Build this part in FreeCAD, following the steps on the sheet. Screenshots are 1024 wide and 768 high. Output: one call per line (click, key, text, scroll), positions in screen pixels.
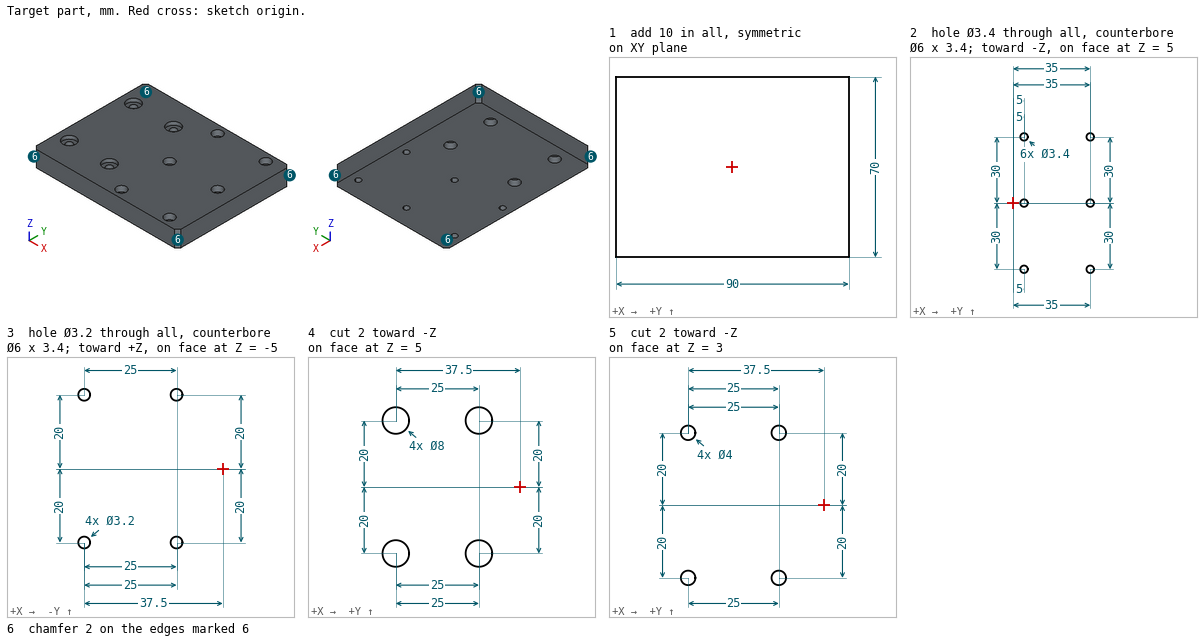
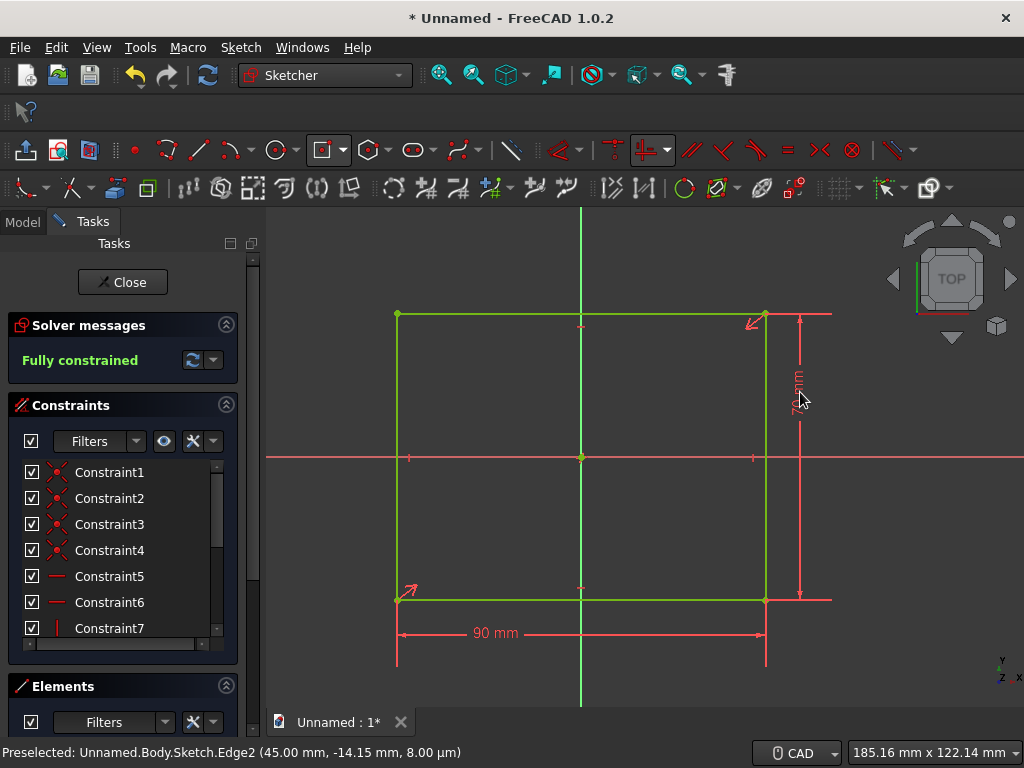
click(123, 282)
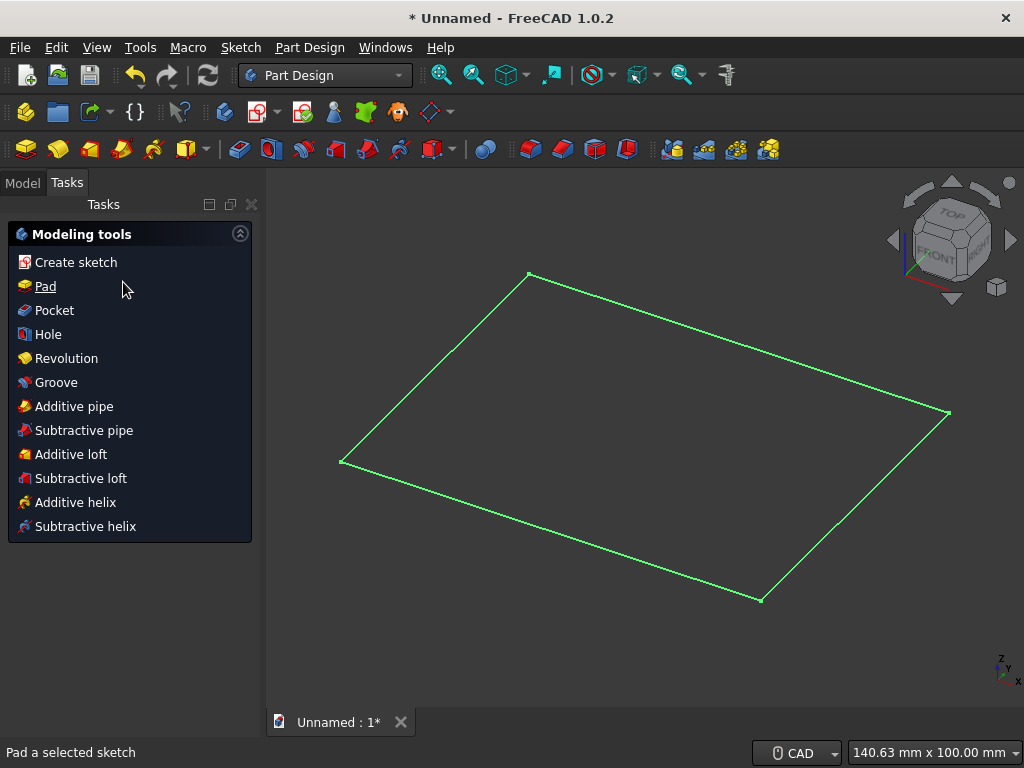
click(26, 150)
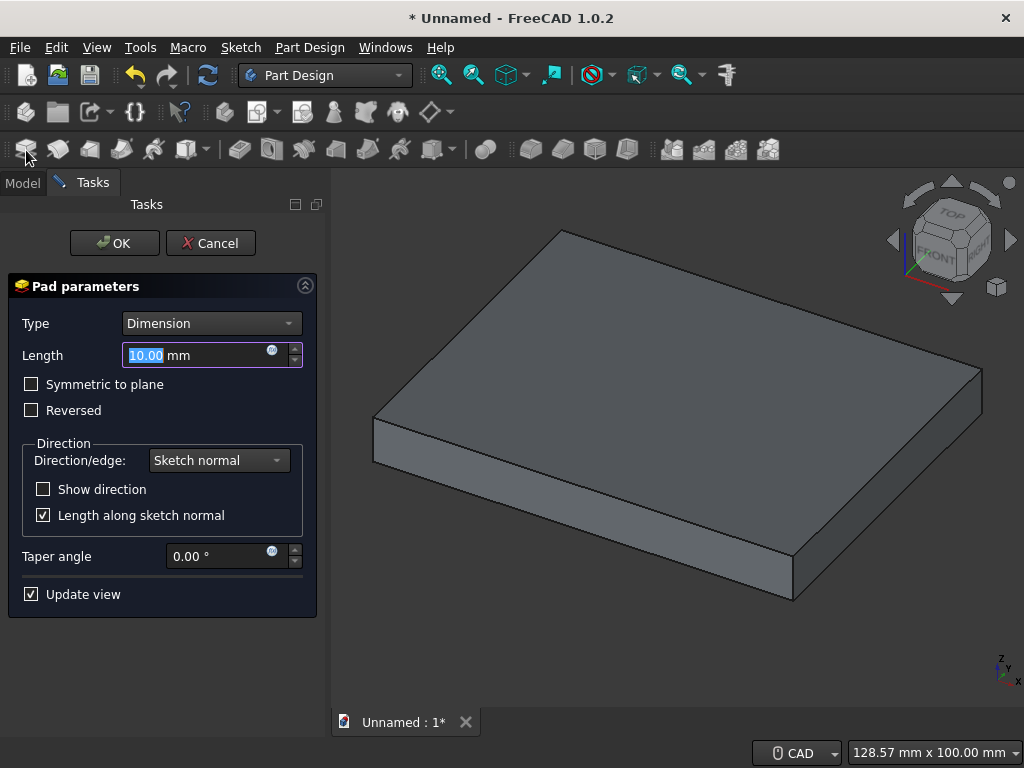
text(10)
key(Tab)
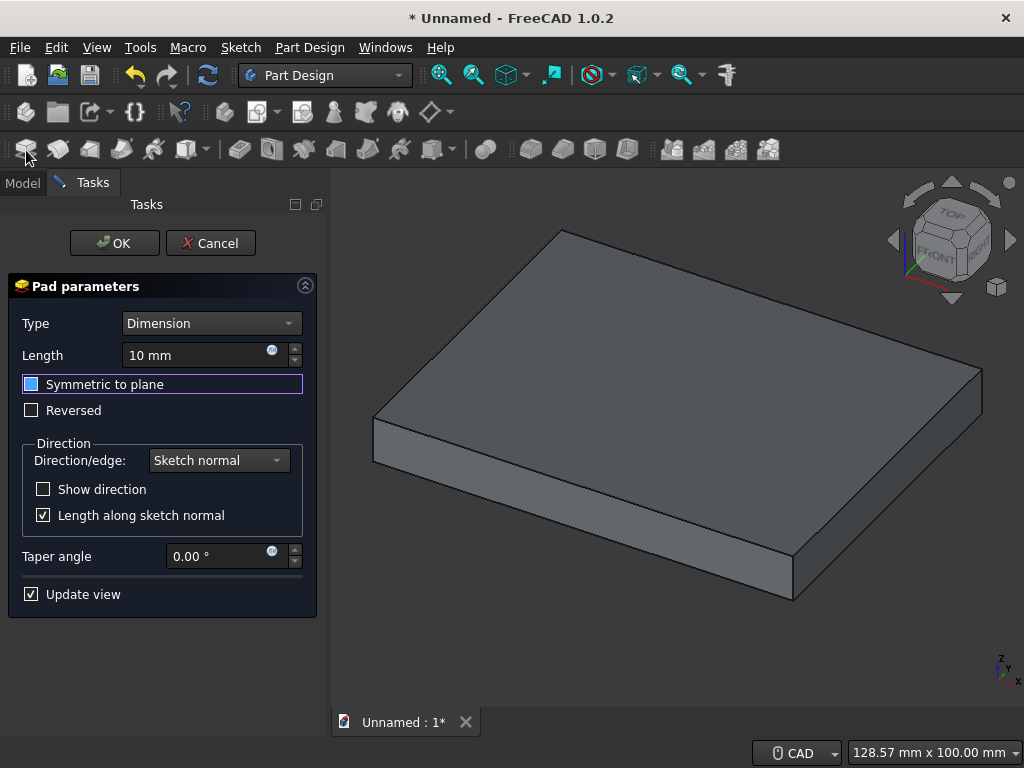
click(30, 384)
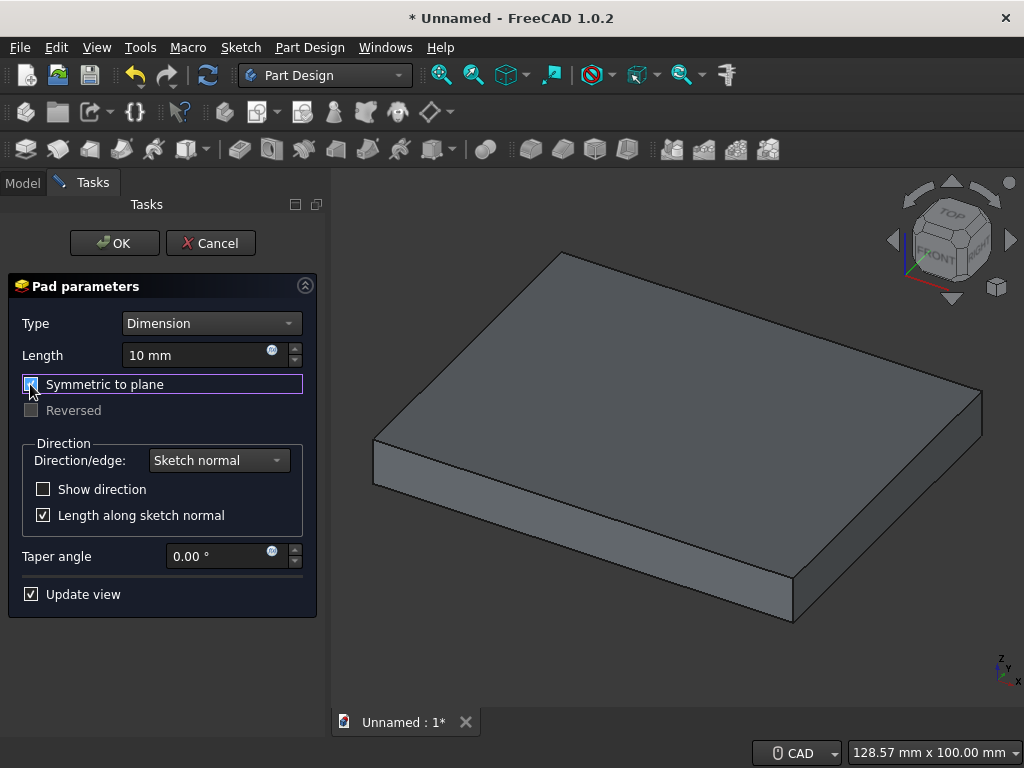
click(115, 243)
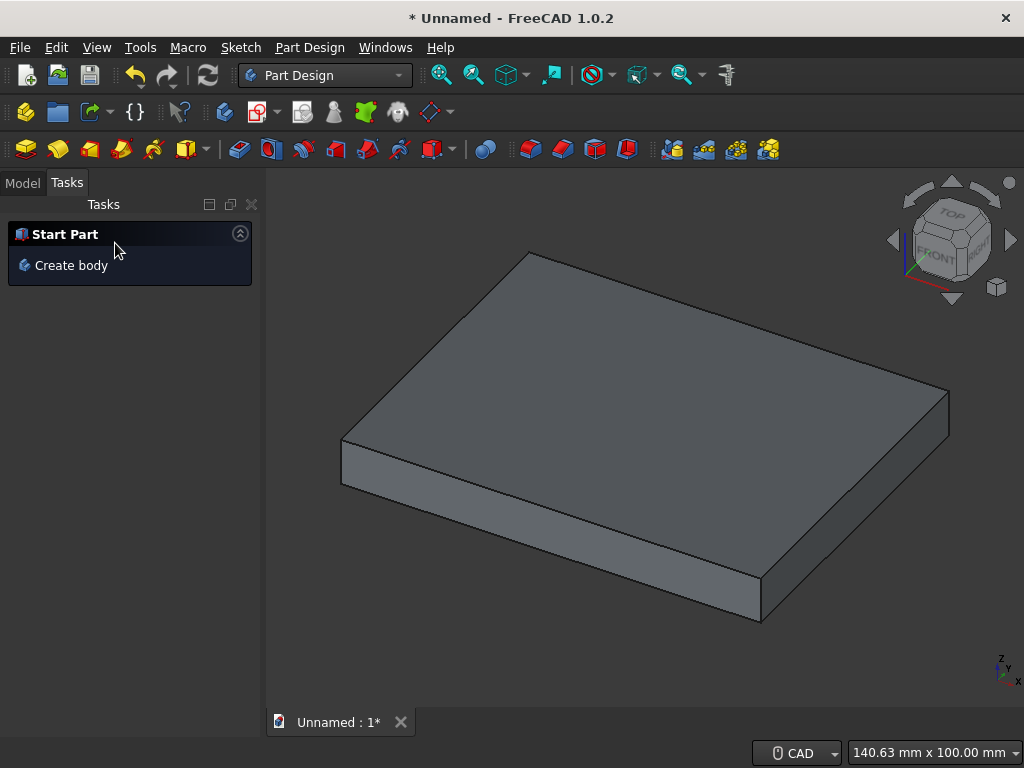
click(645, 414)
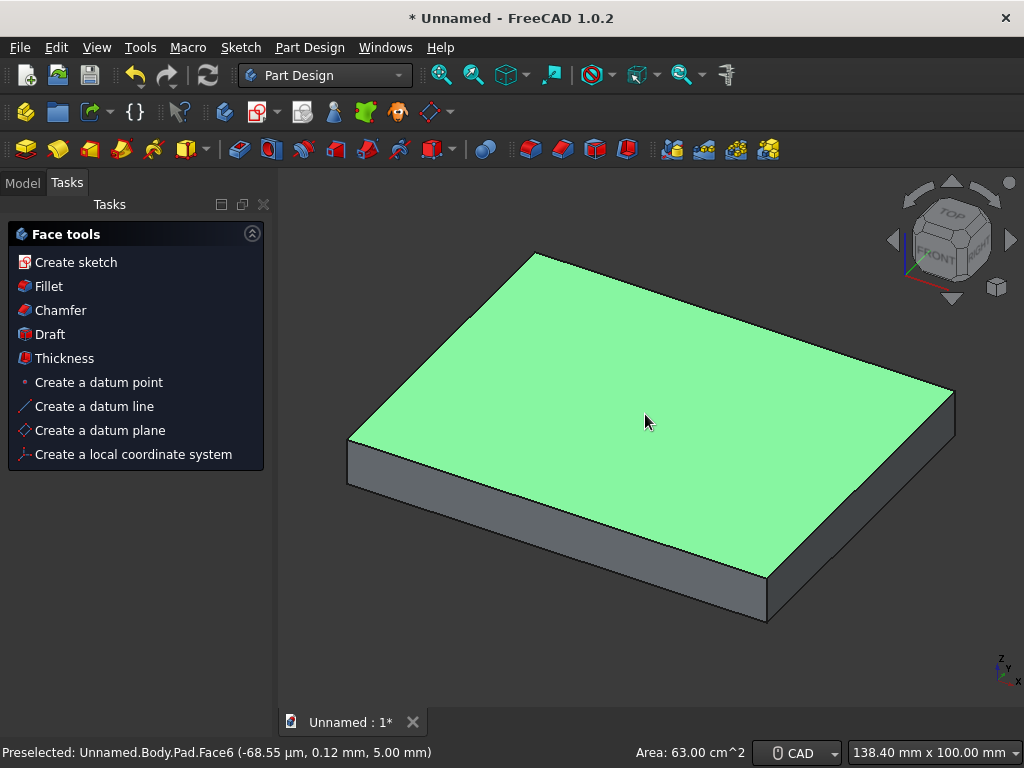
click(258, 112)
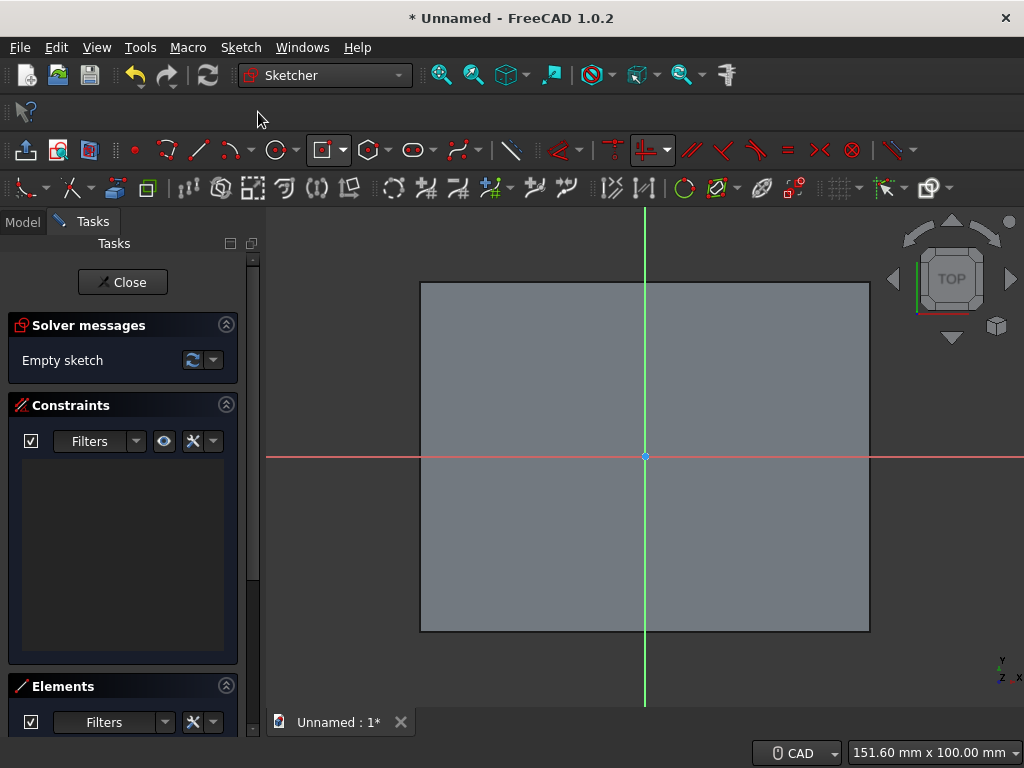
click(276, 150)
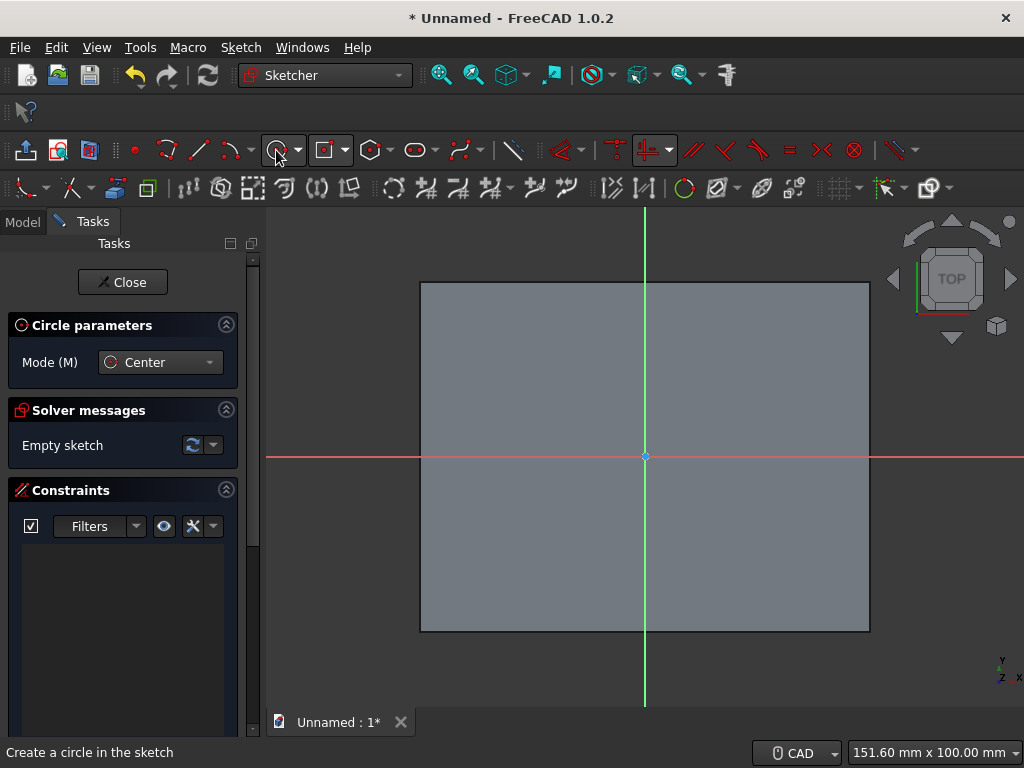
scroll(670, 307, up, 5)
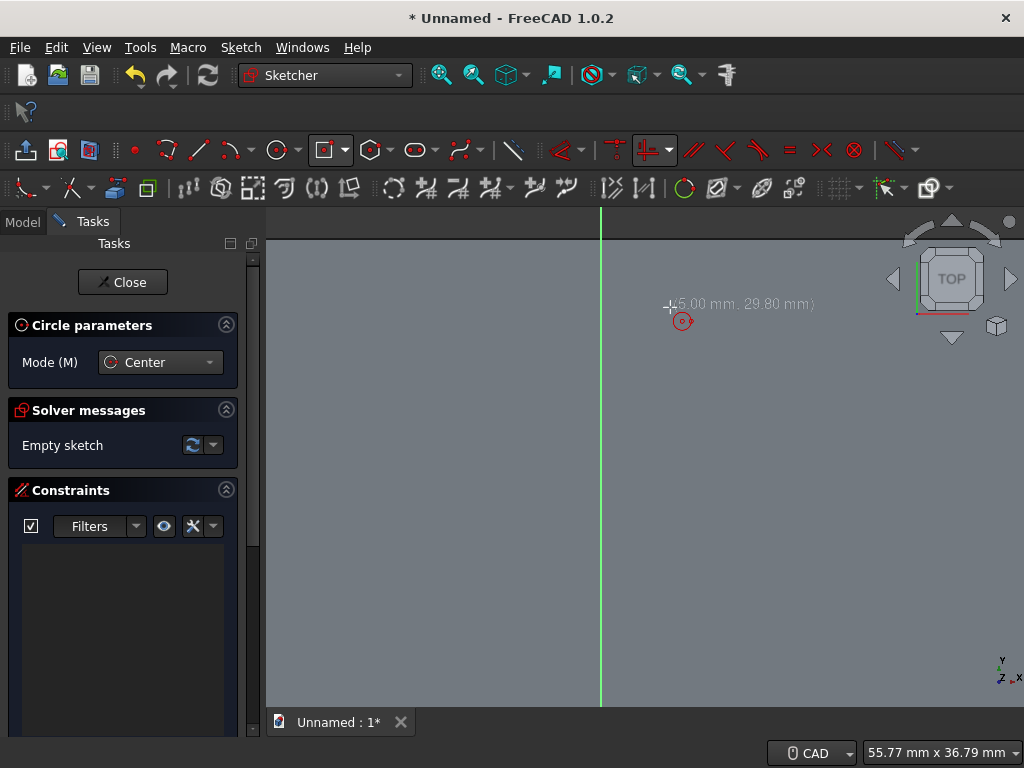
click(669, 307)
click(685, 290)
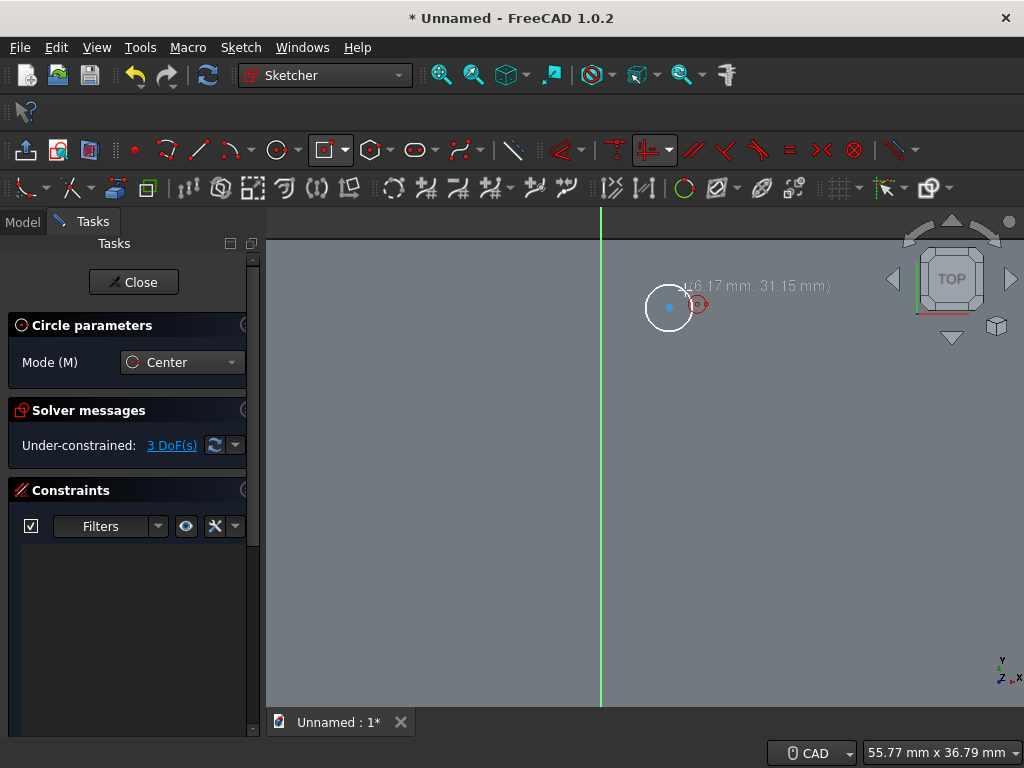
scroll(417, 307, down, 5)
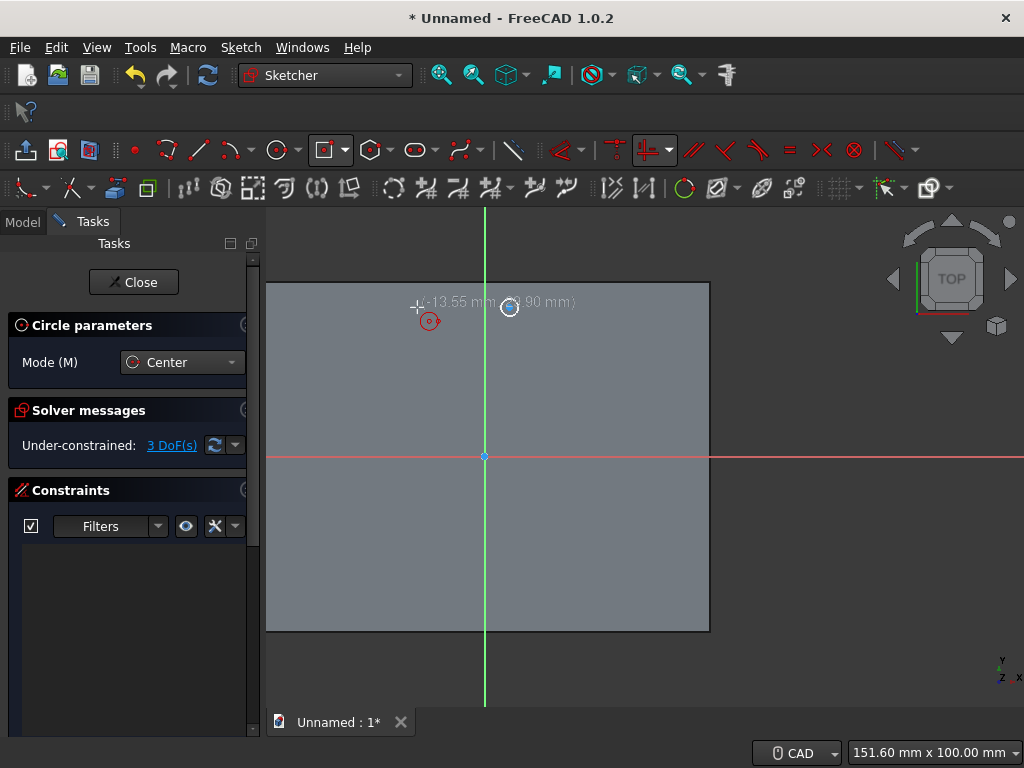
scroll(510, 457, up, 5)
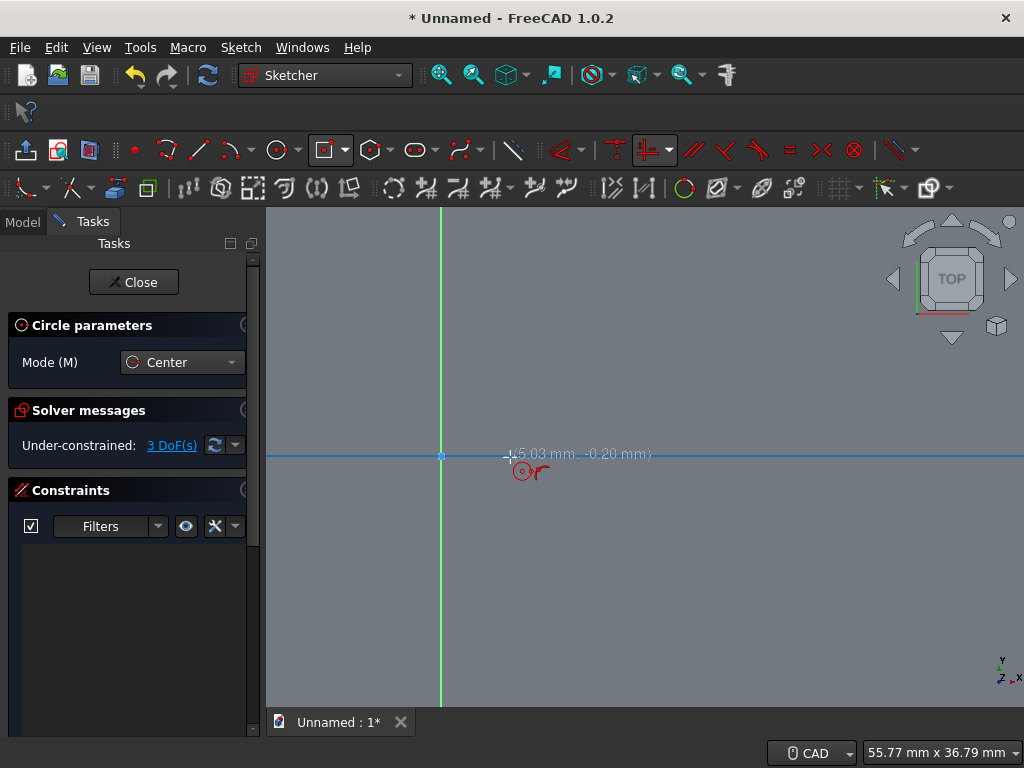
click(509, 456)
click(525, 440)